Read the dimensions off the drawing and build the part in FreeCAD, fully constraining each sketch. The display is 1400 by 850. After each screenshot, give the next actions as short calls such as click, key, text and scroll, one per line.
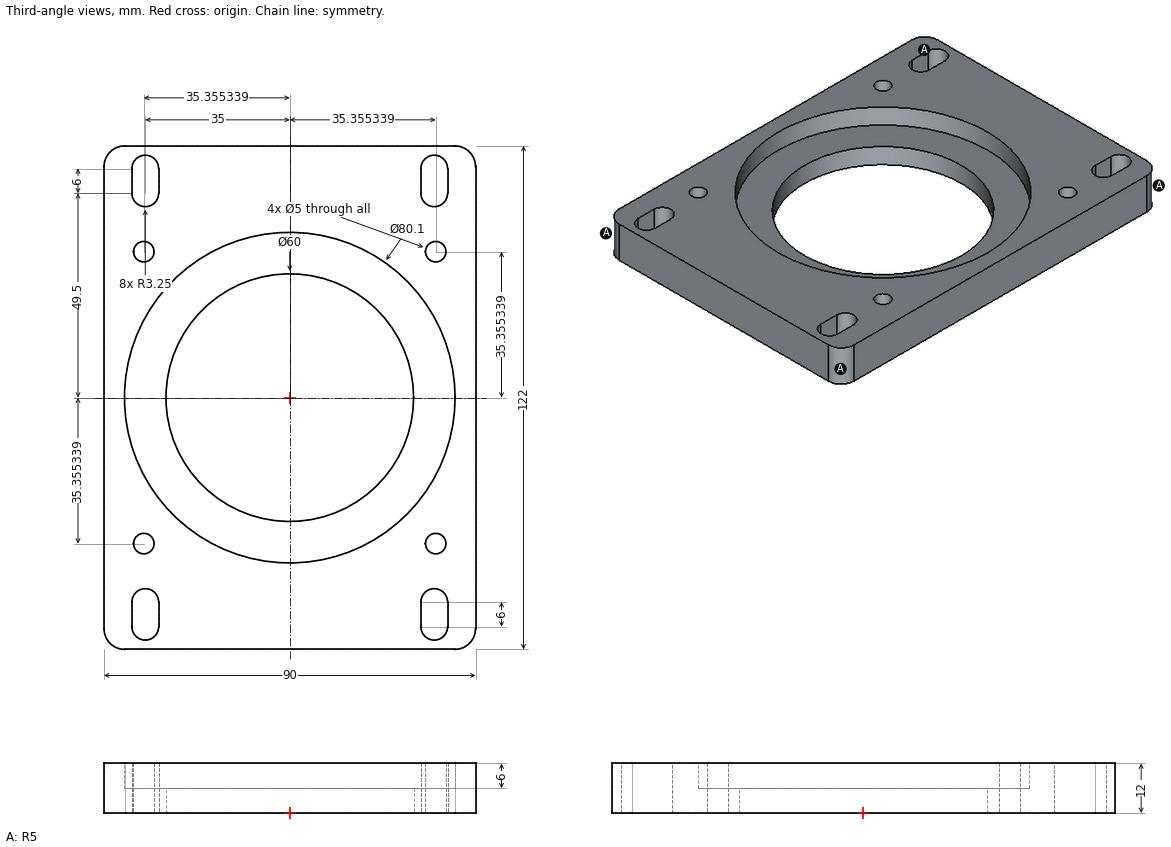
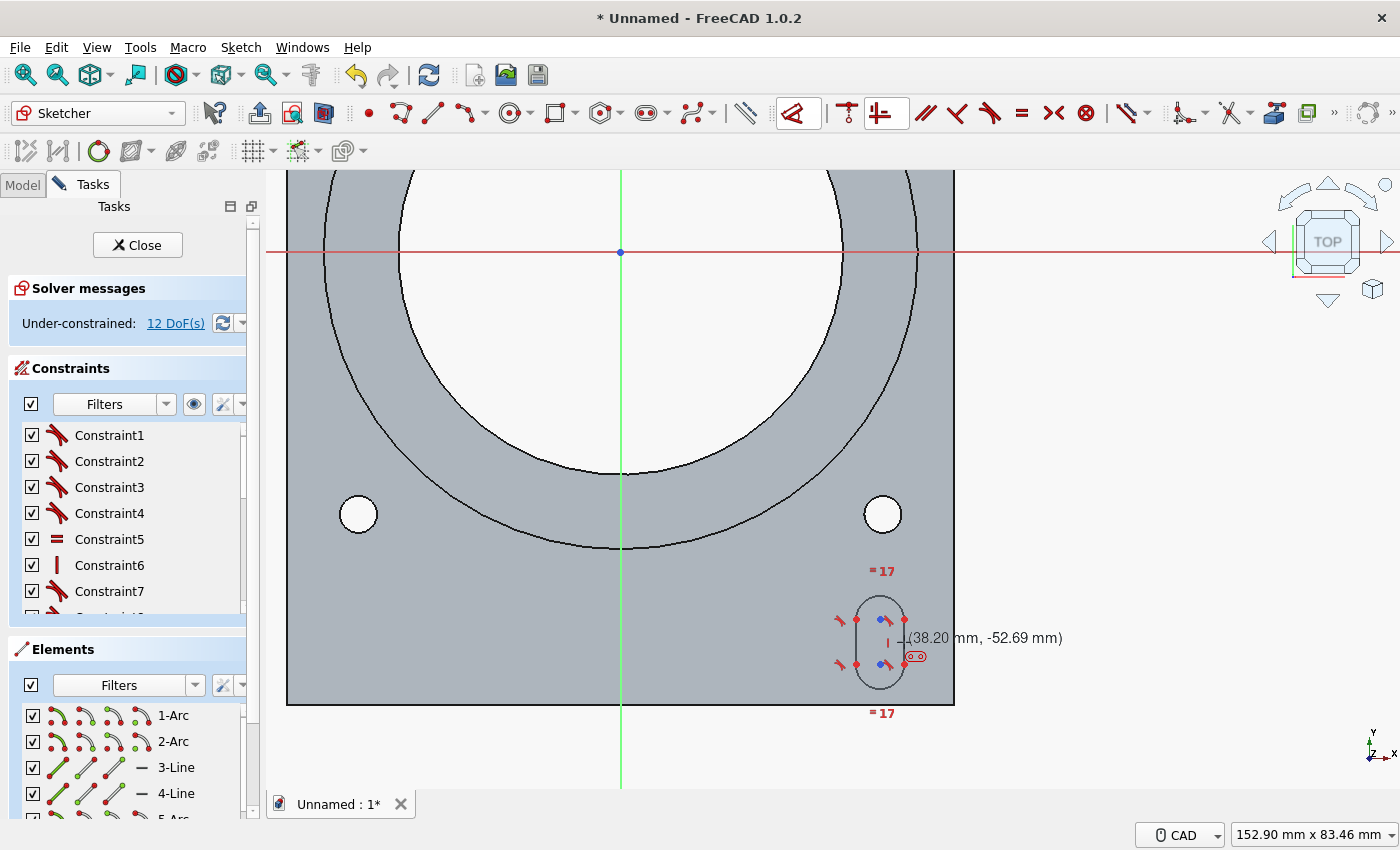
click(361, 664)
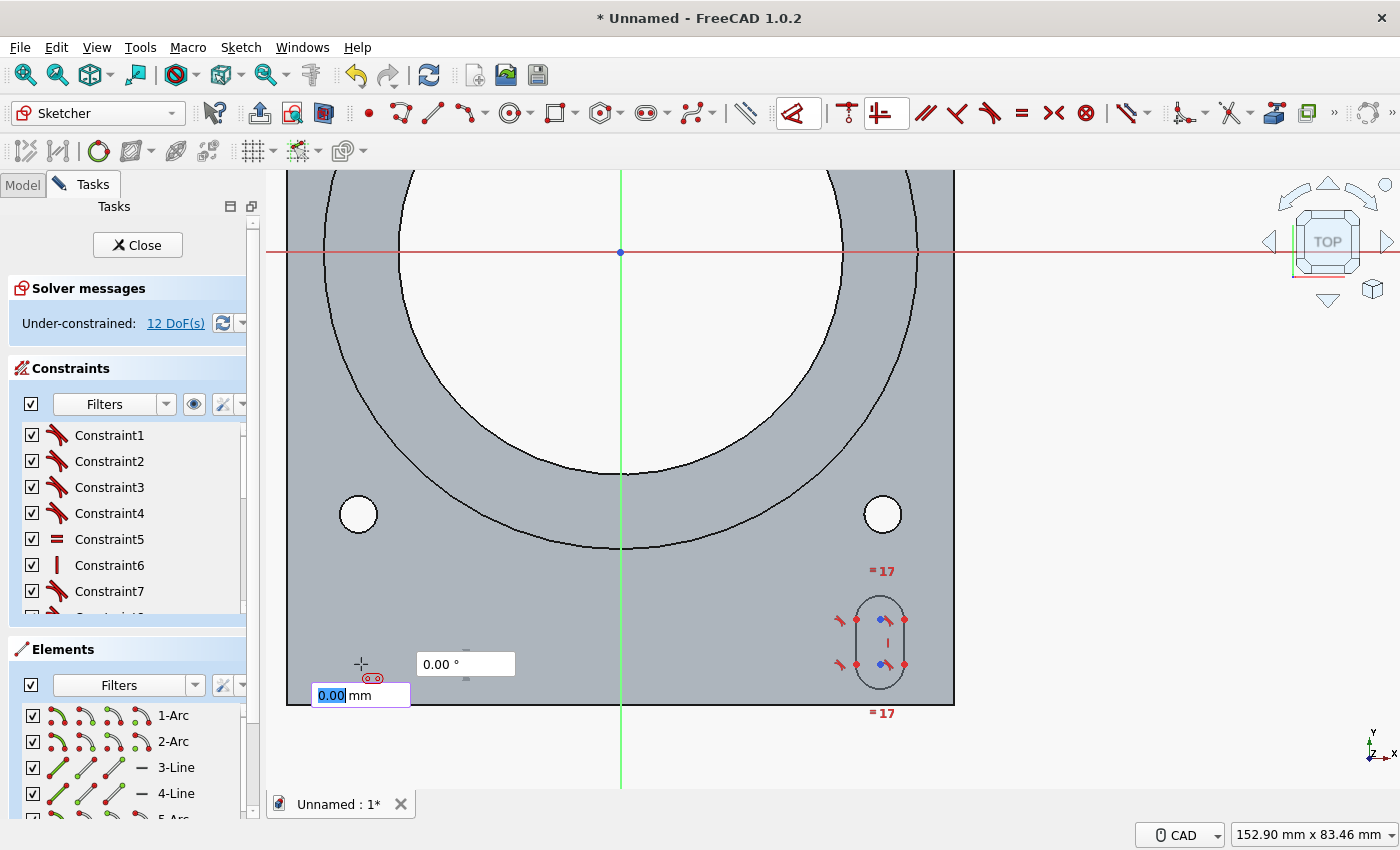
click(361, 619)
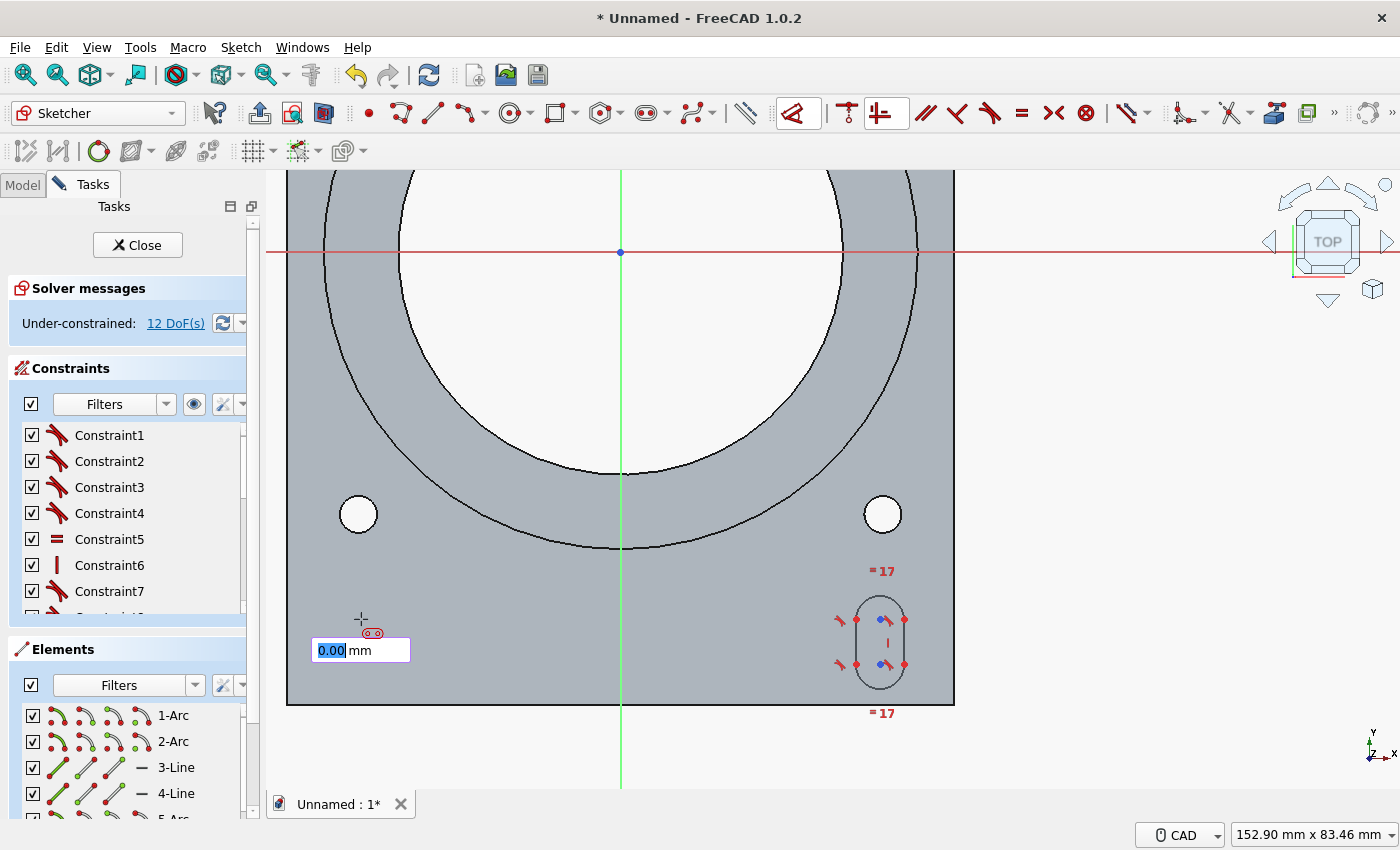
click(337, 642)
key(Escape)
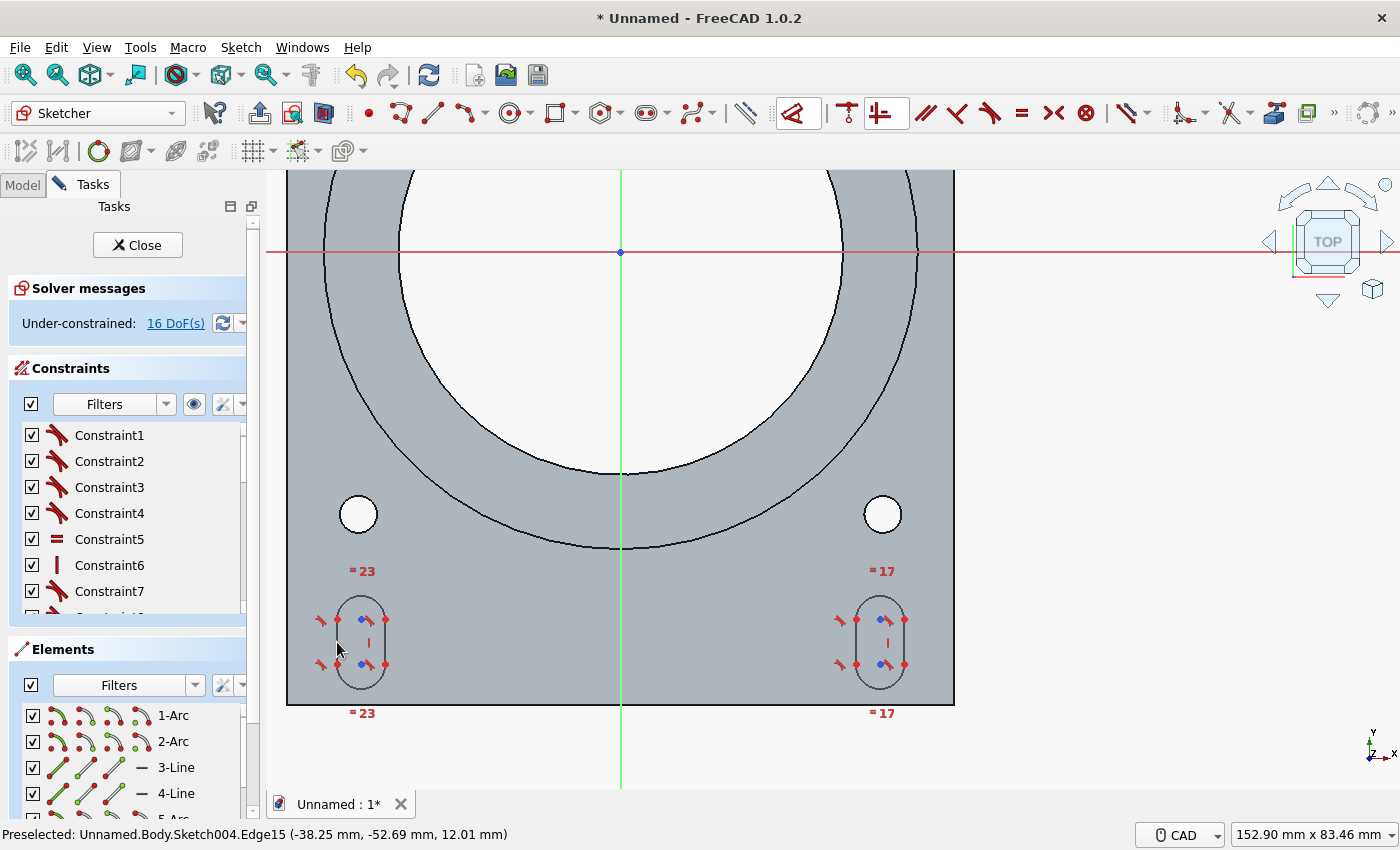
scroll(882, 665, down, 4)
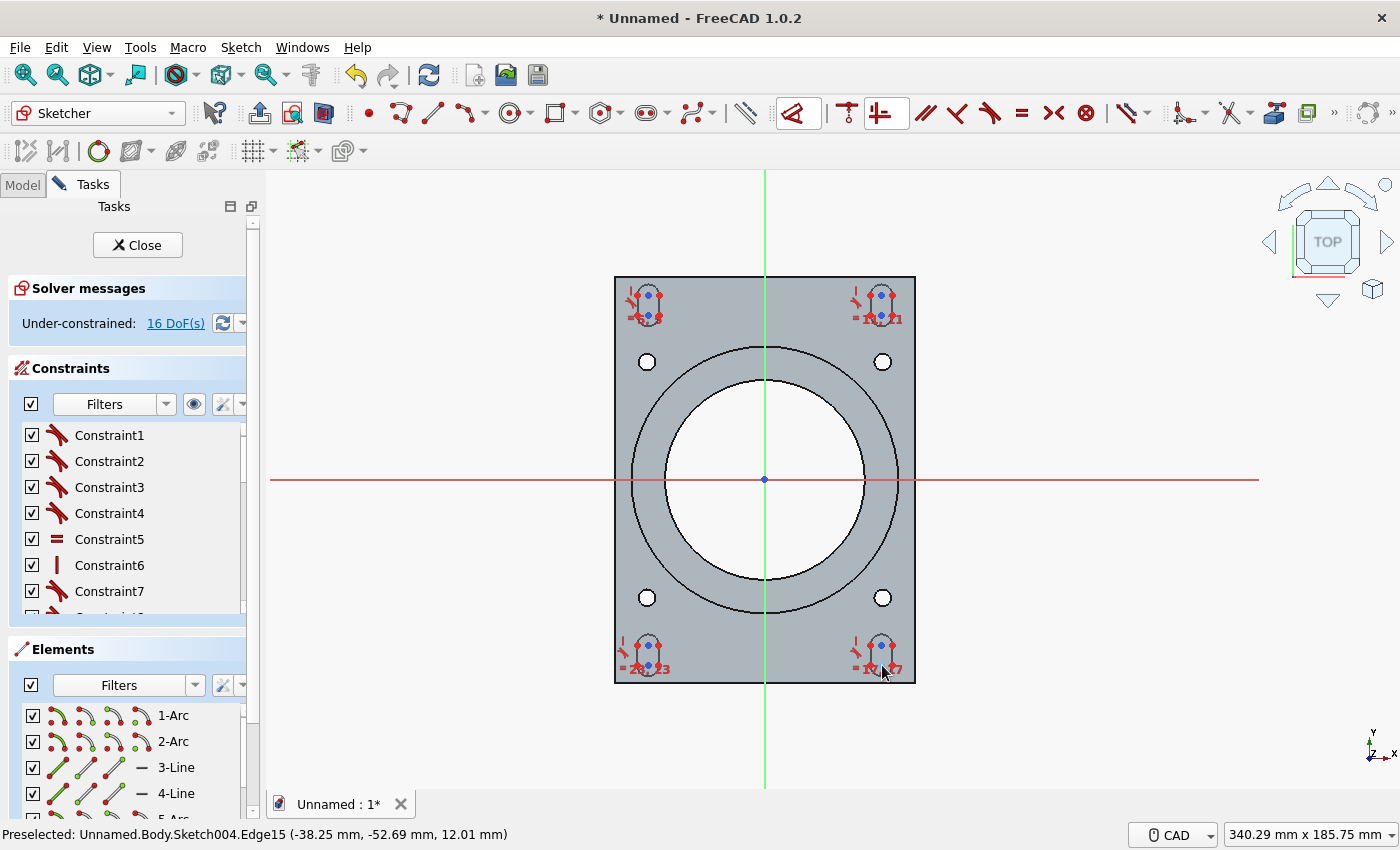
scroll(642, 324, up, 2)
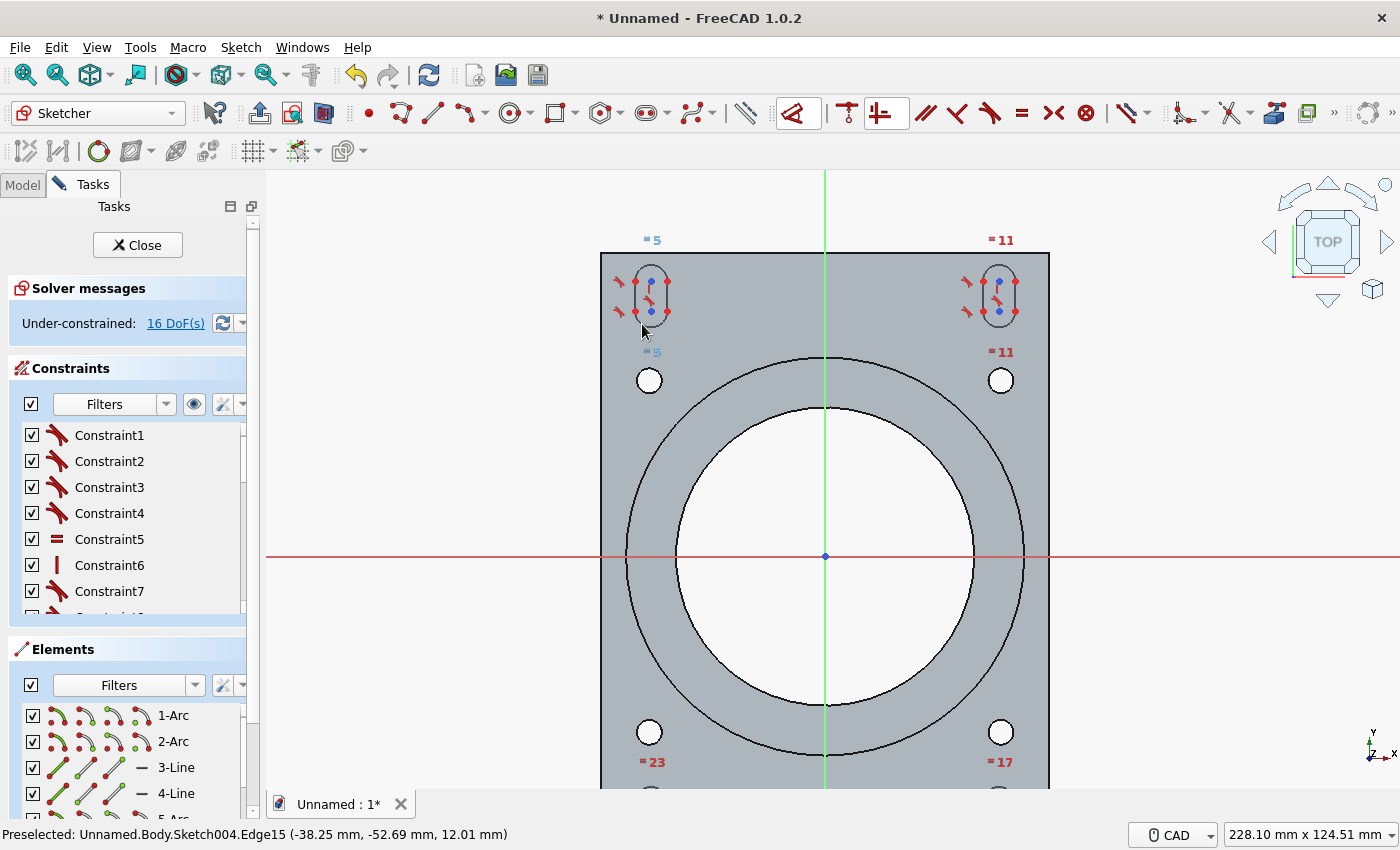
click(642, 324)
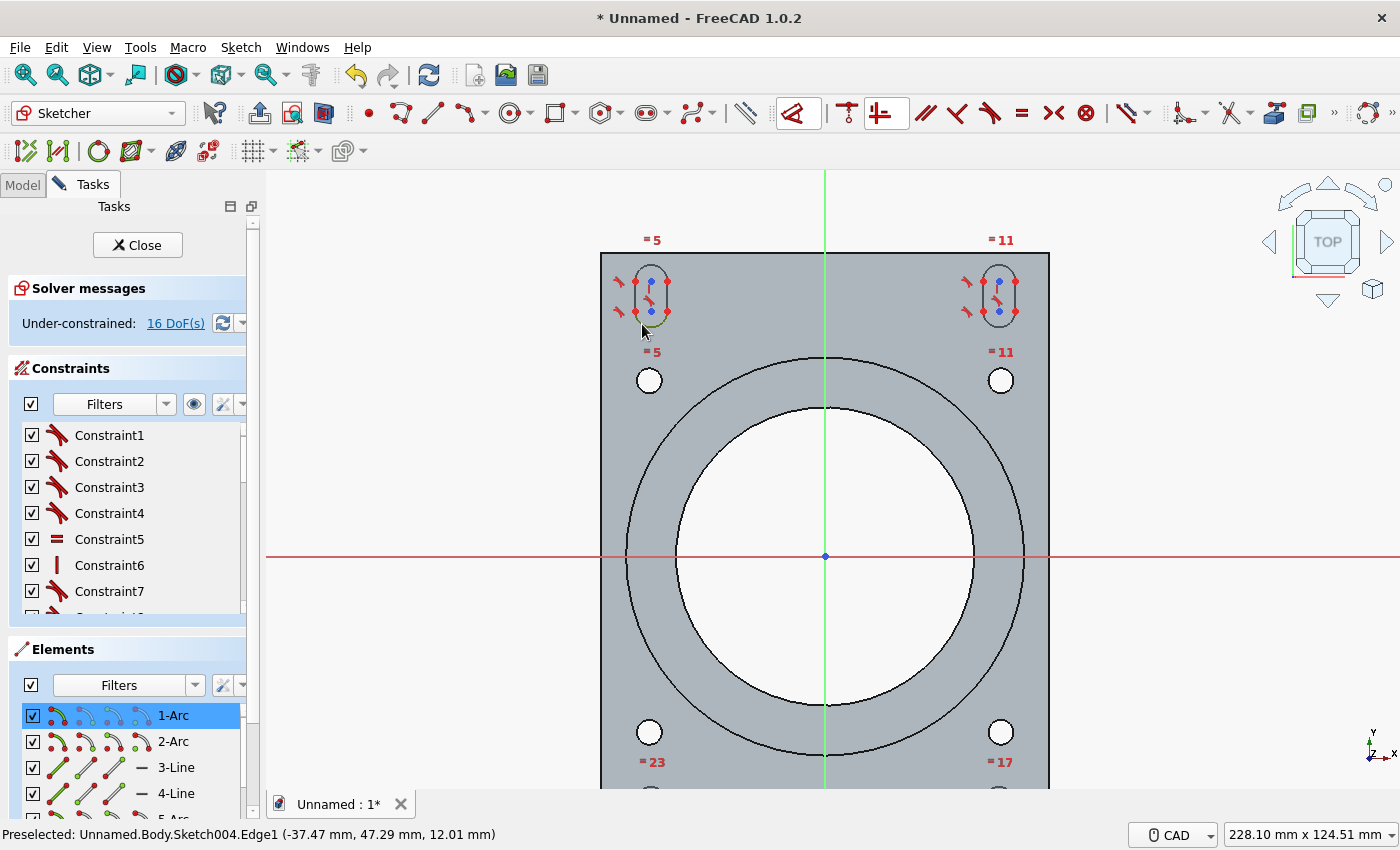
click(990, 324)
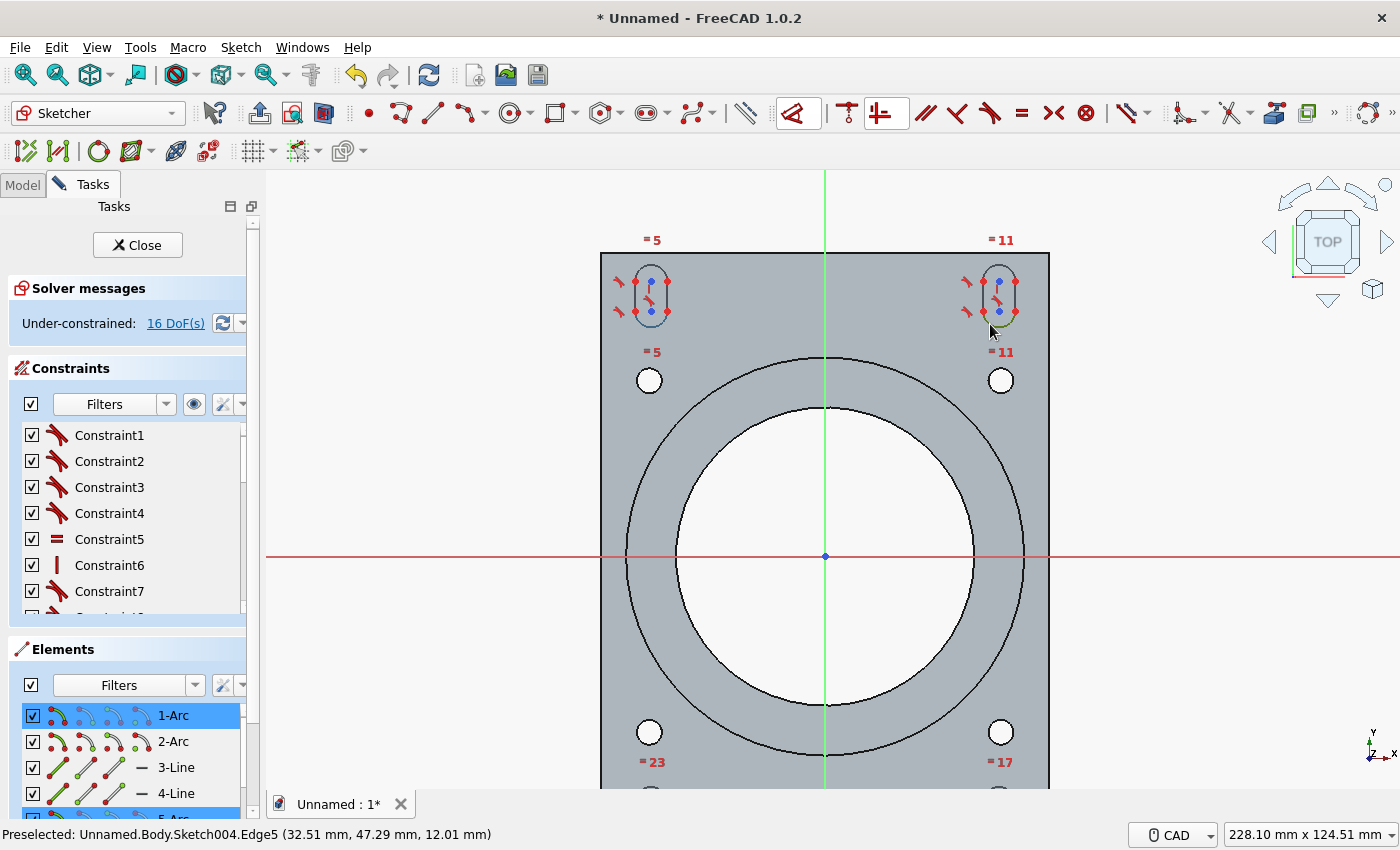
scroll(641, 323, down, 2)